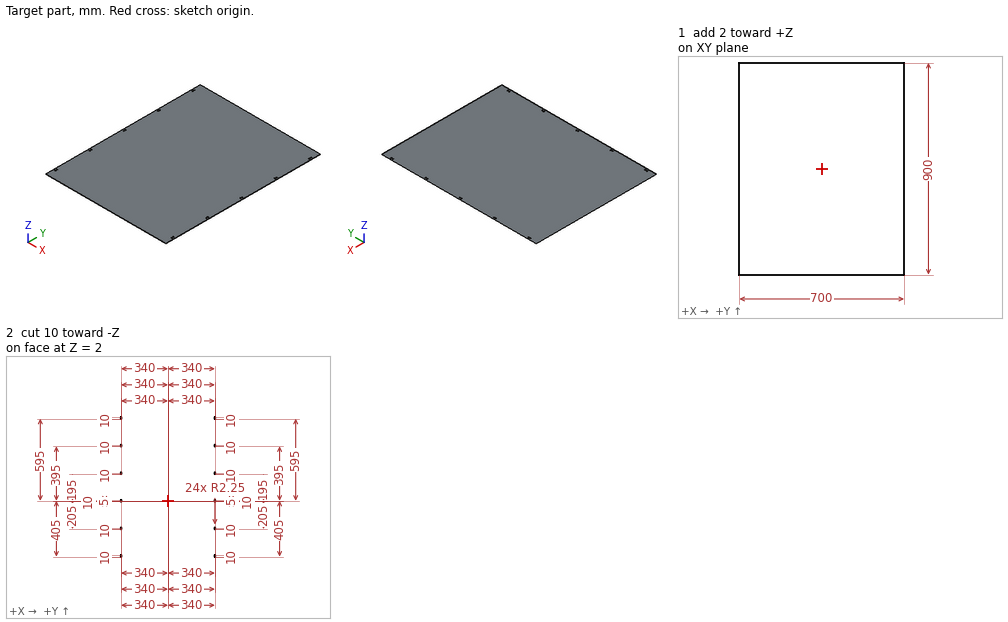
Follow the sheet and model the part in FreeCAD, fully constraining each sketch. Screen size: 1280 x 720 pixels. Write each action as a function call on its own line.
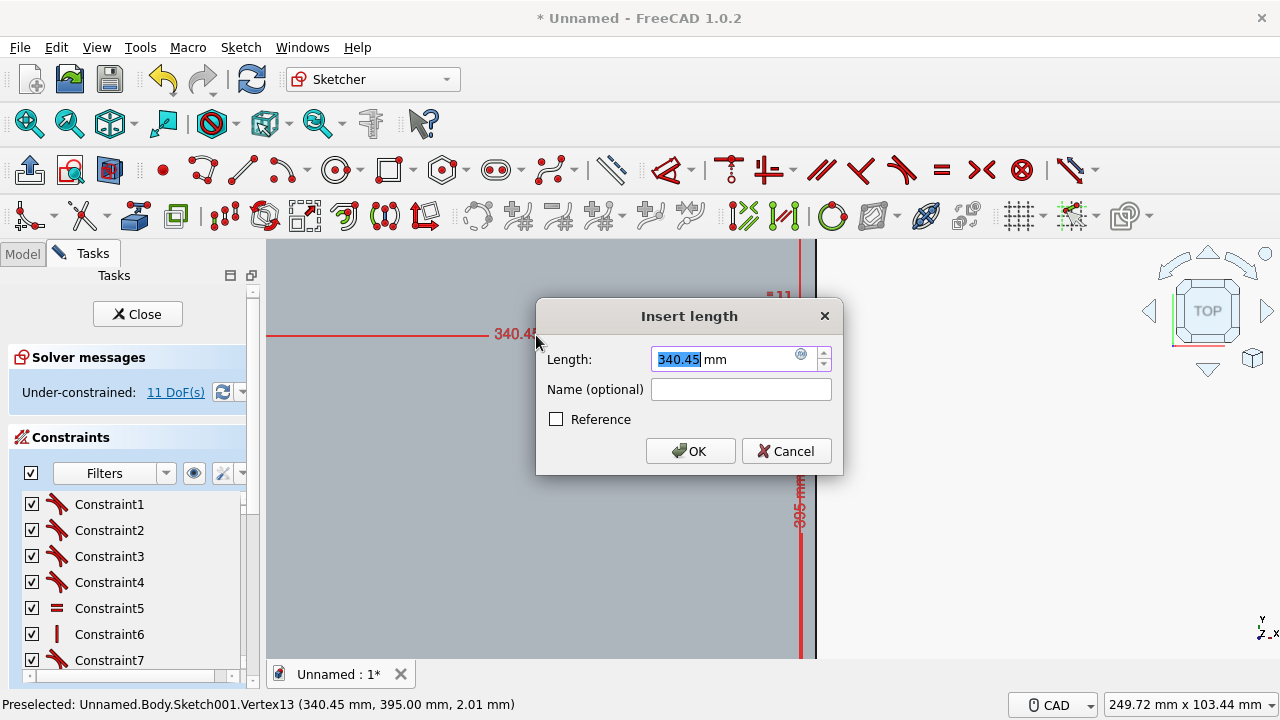
text(340)
key(Return)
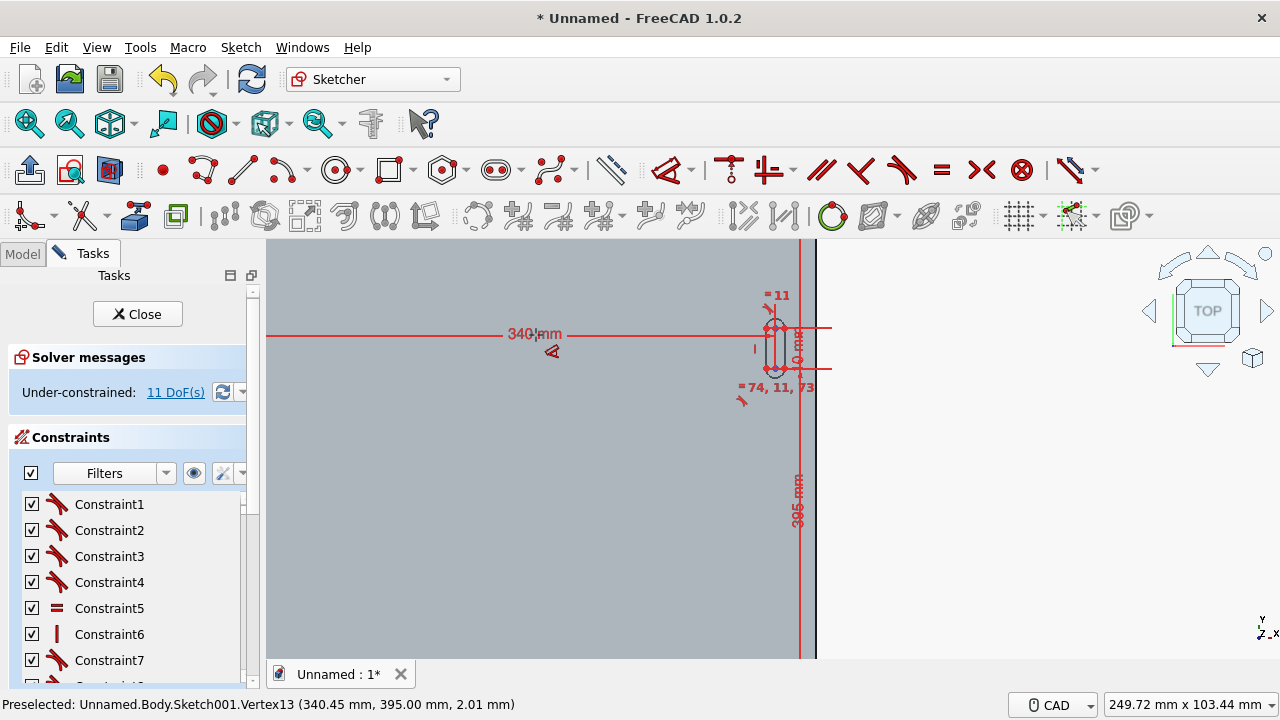
scroll(789, 377, down, 14)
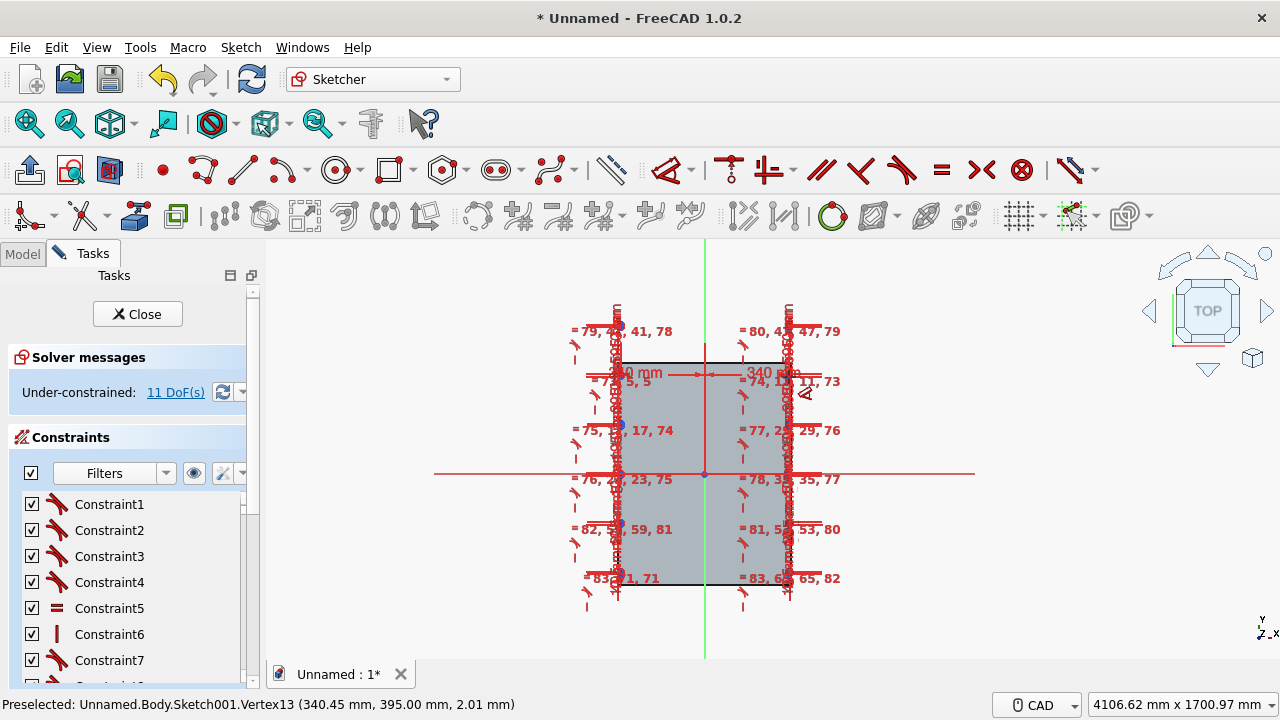
scroll(621, 426, up, 14)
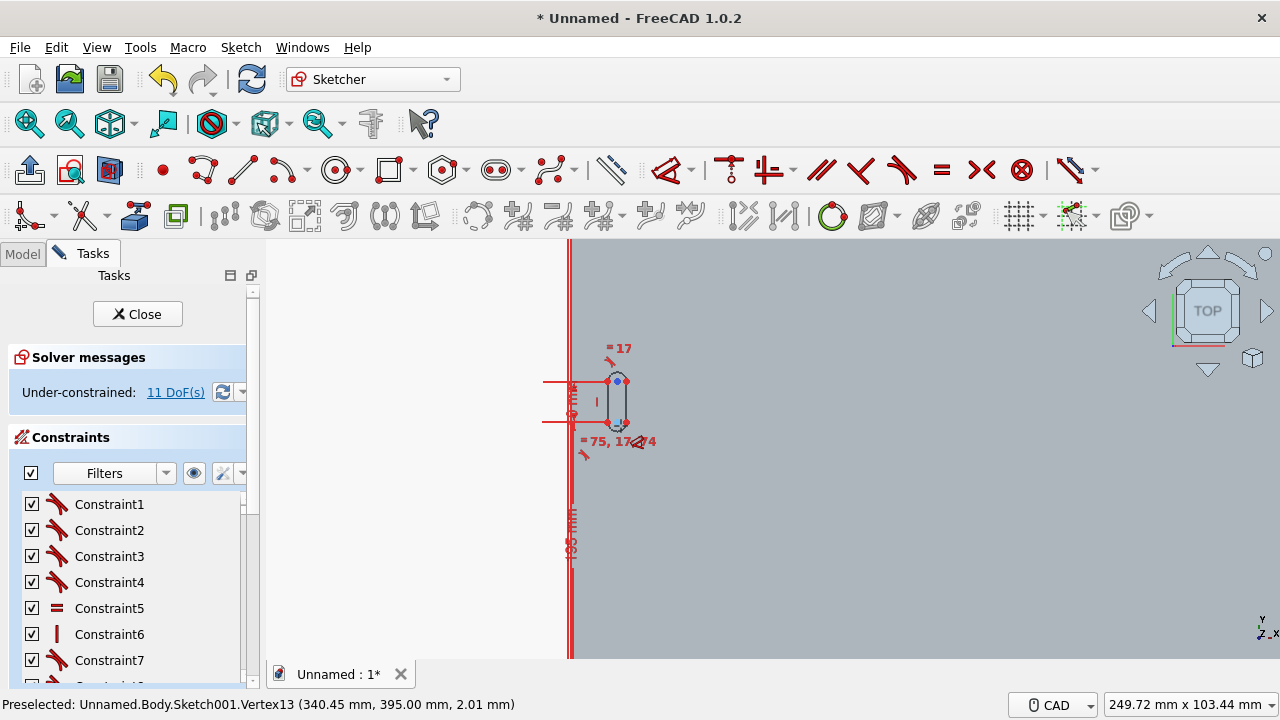
click(617, 422)
click(866, 388)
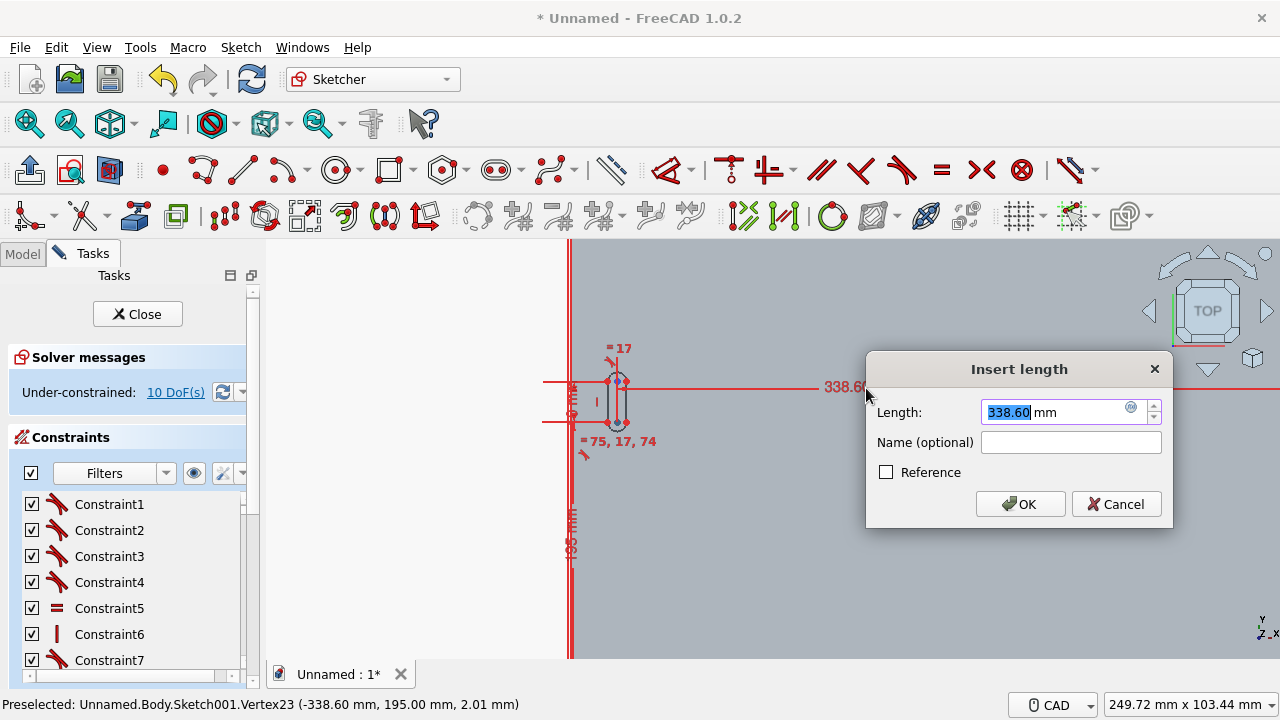
text(340)
key(Return)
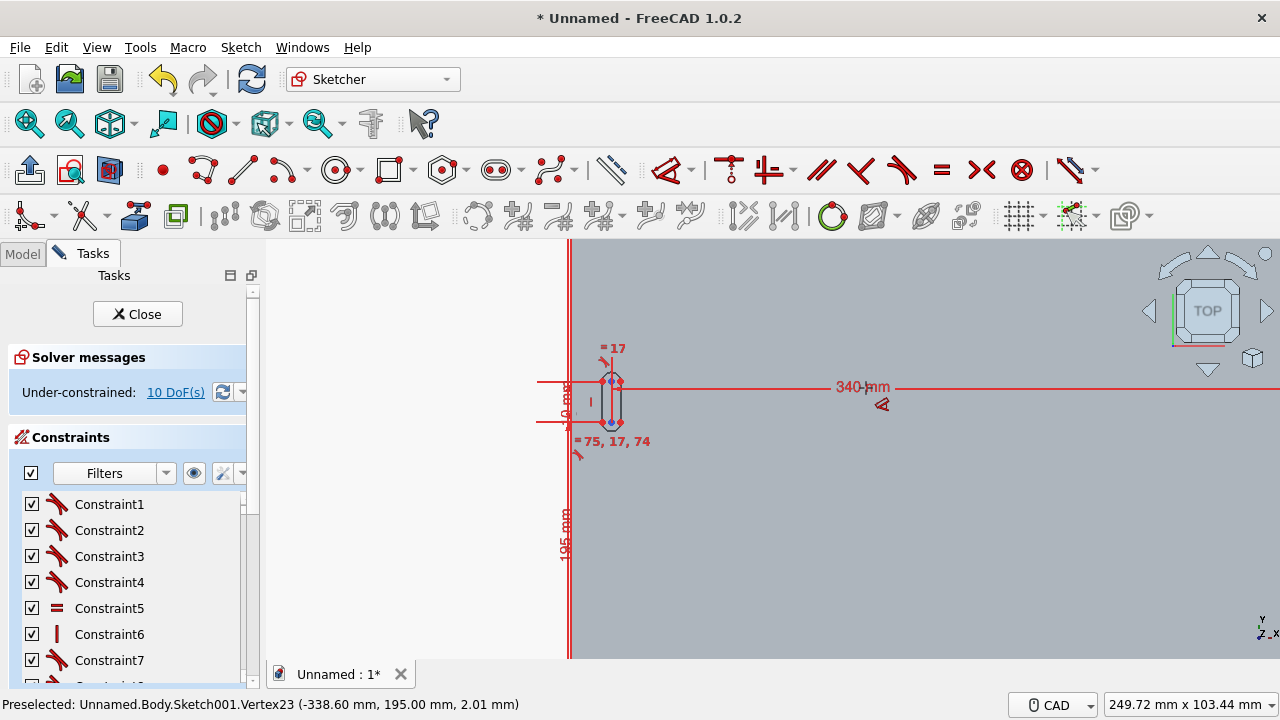
scroll(621, 426, down, 14)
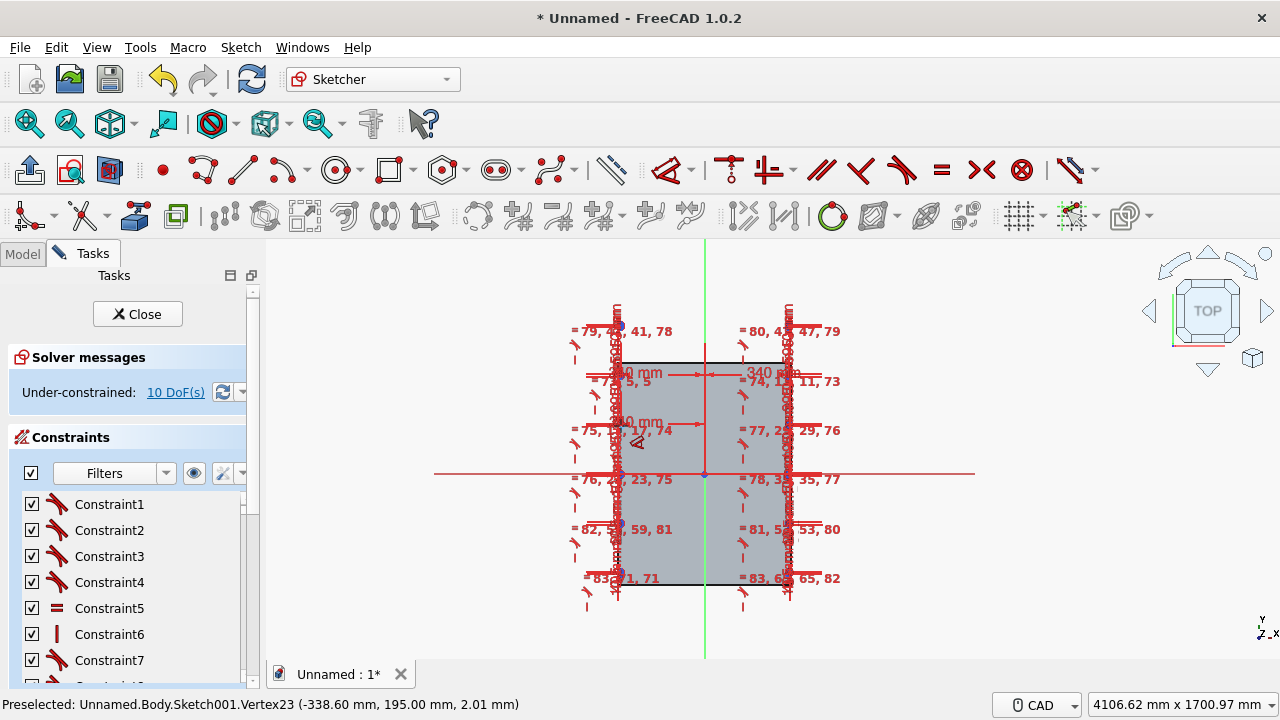
scroll(621, 476, up, 14)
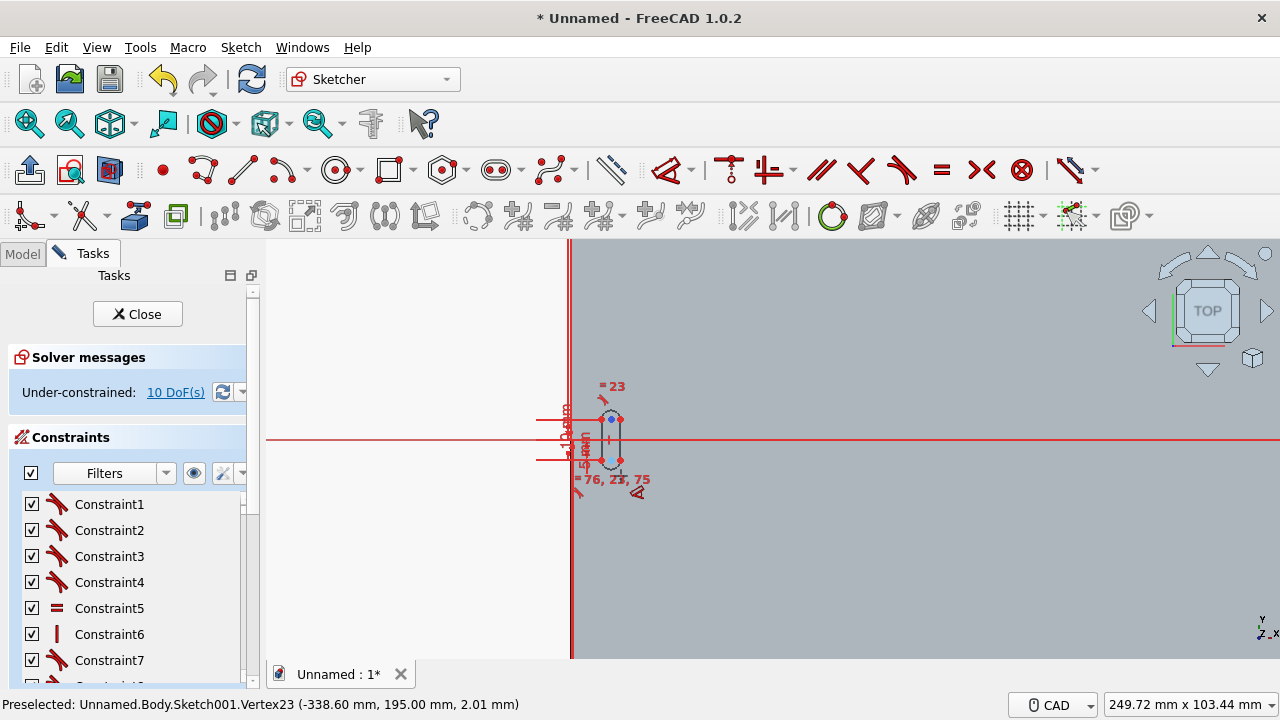
click(611, 460)
click(863, 494)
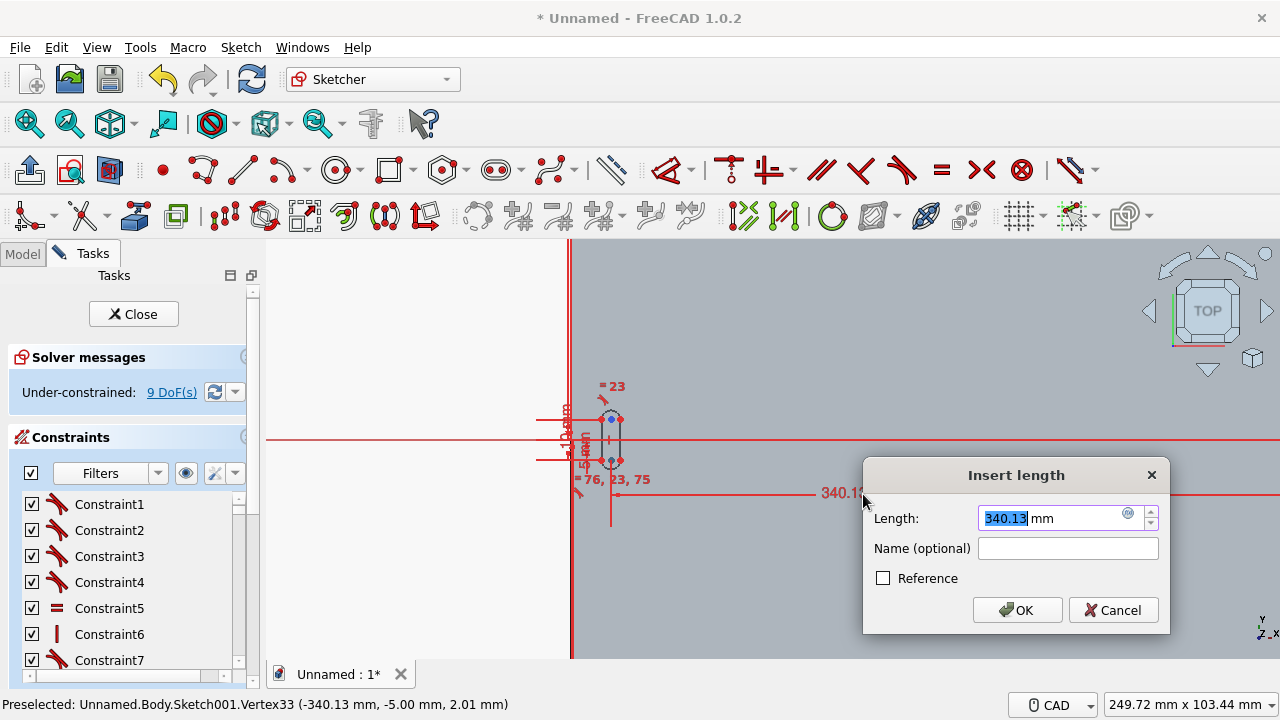
text(340)
key(Return)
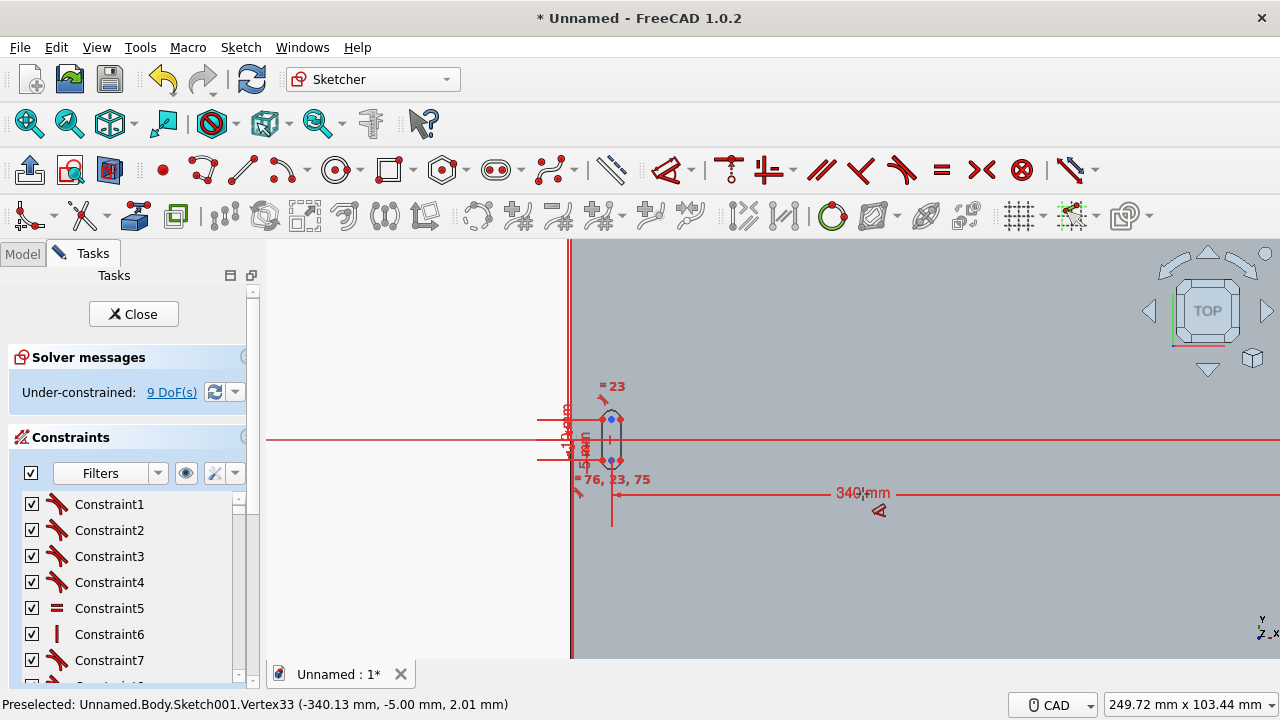
scroll(621, 476, down, 14)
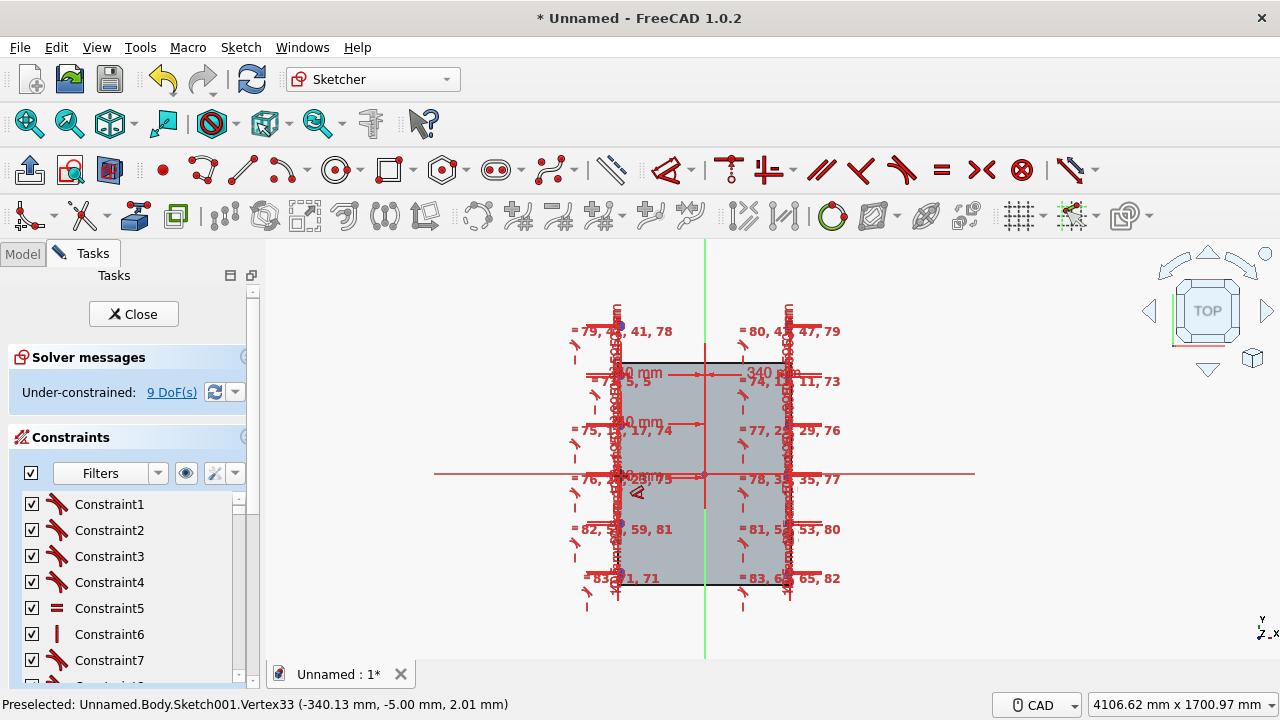
scroll(789, 426, up, 14)